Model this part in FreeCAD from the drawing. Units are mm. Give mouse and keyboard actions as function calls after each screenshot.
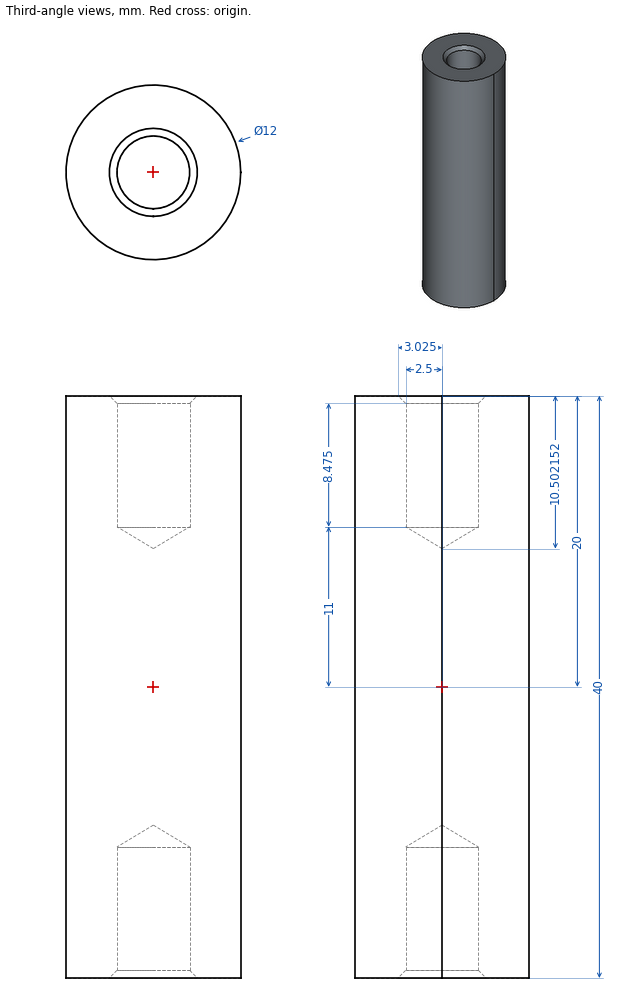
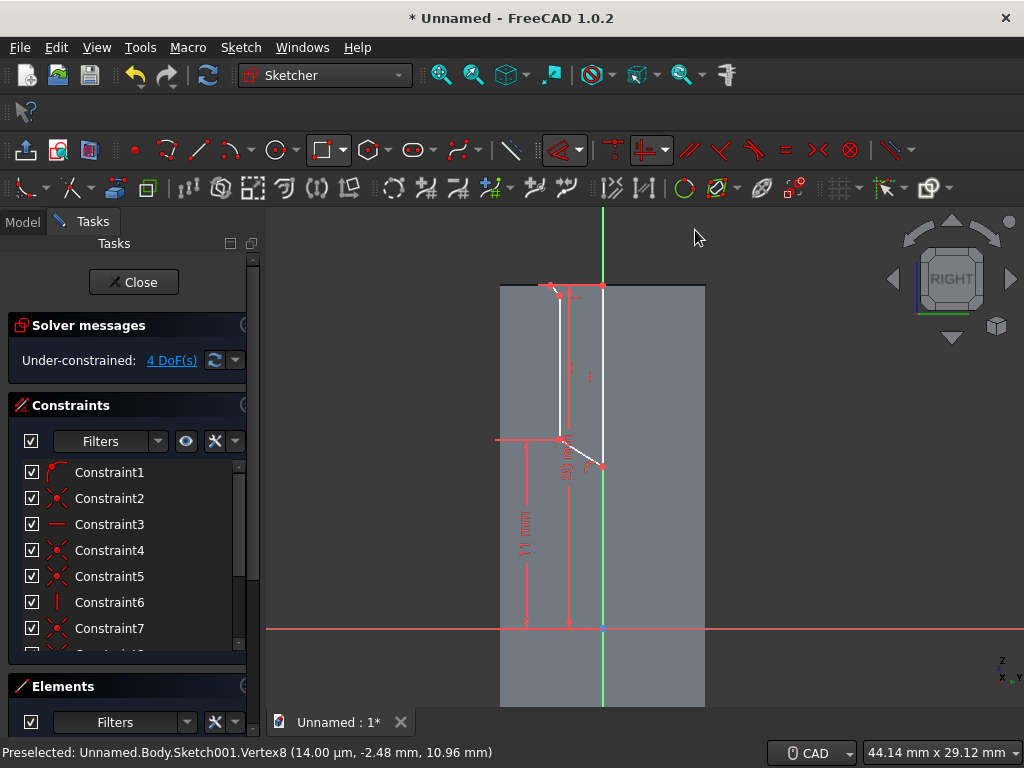
click(560, 295)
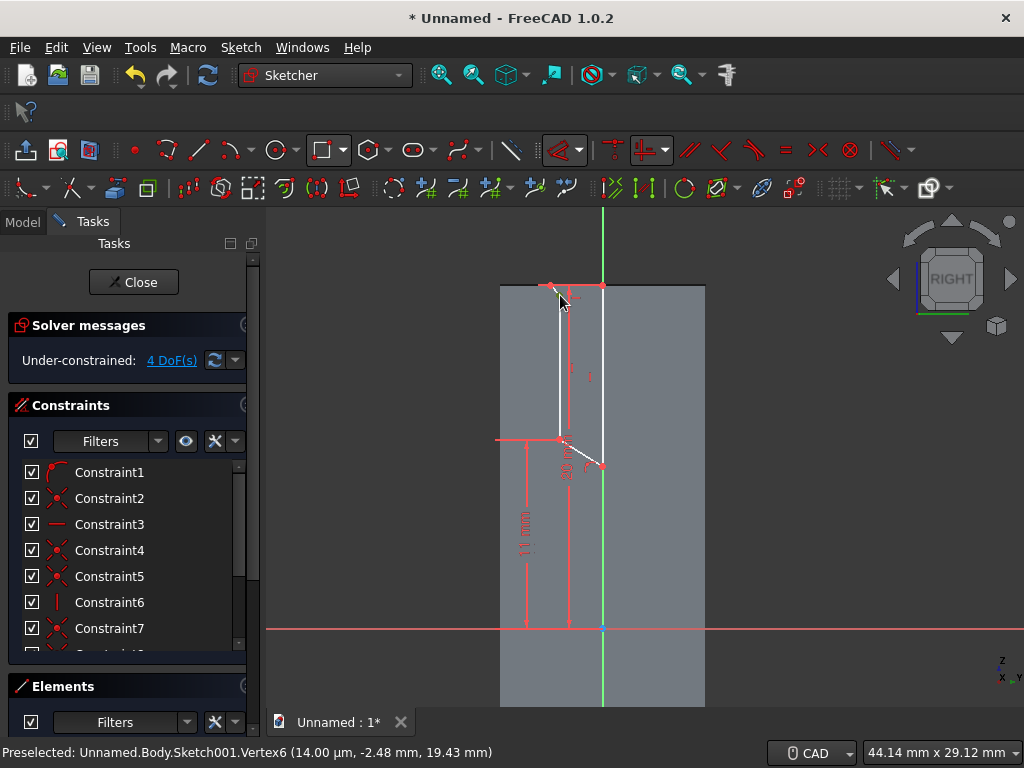
key(l)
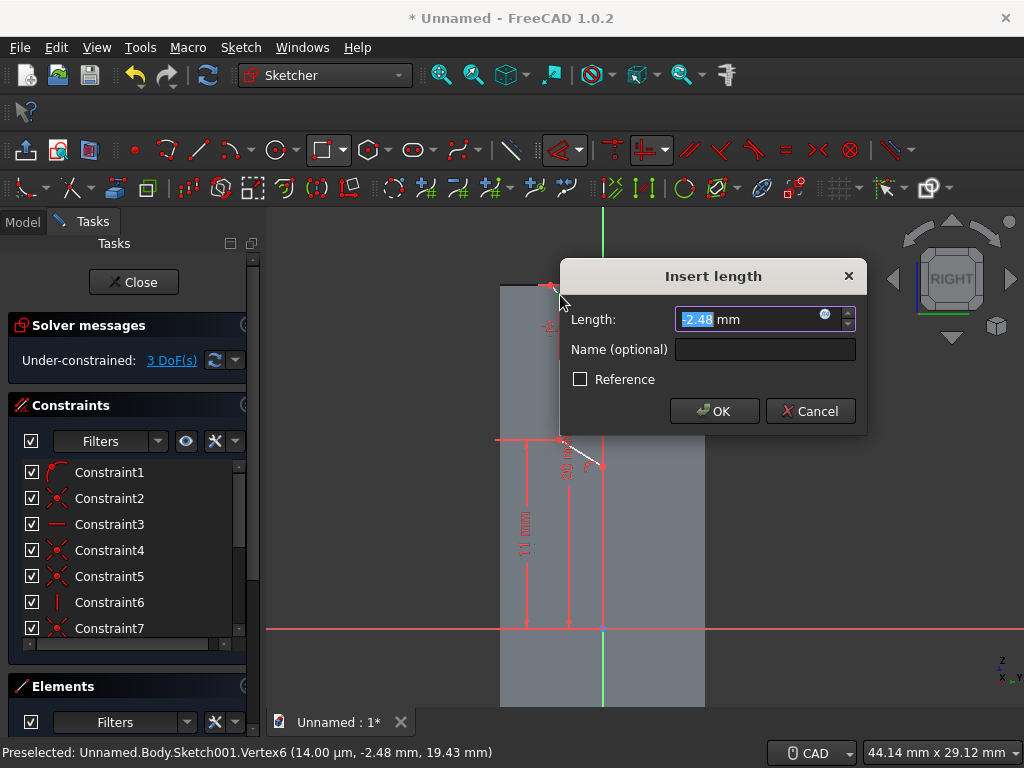
text(-2.5)
key(Return)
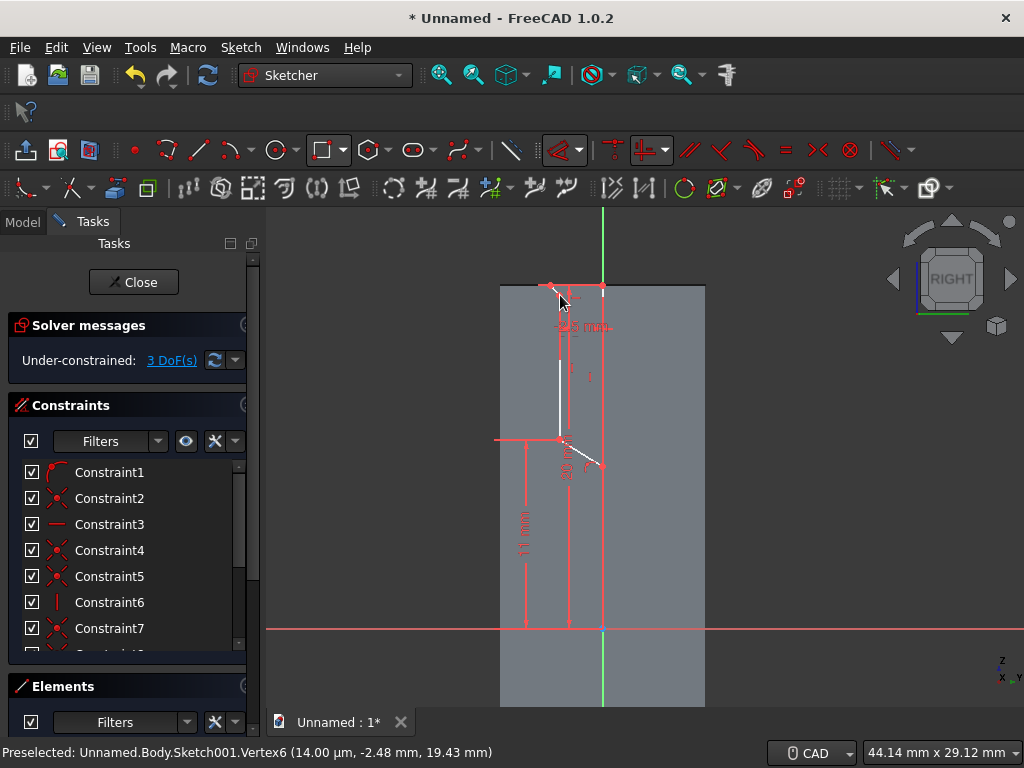
click(587, 285)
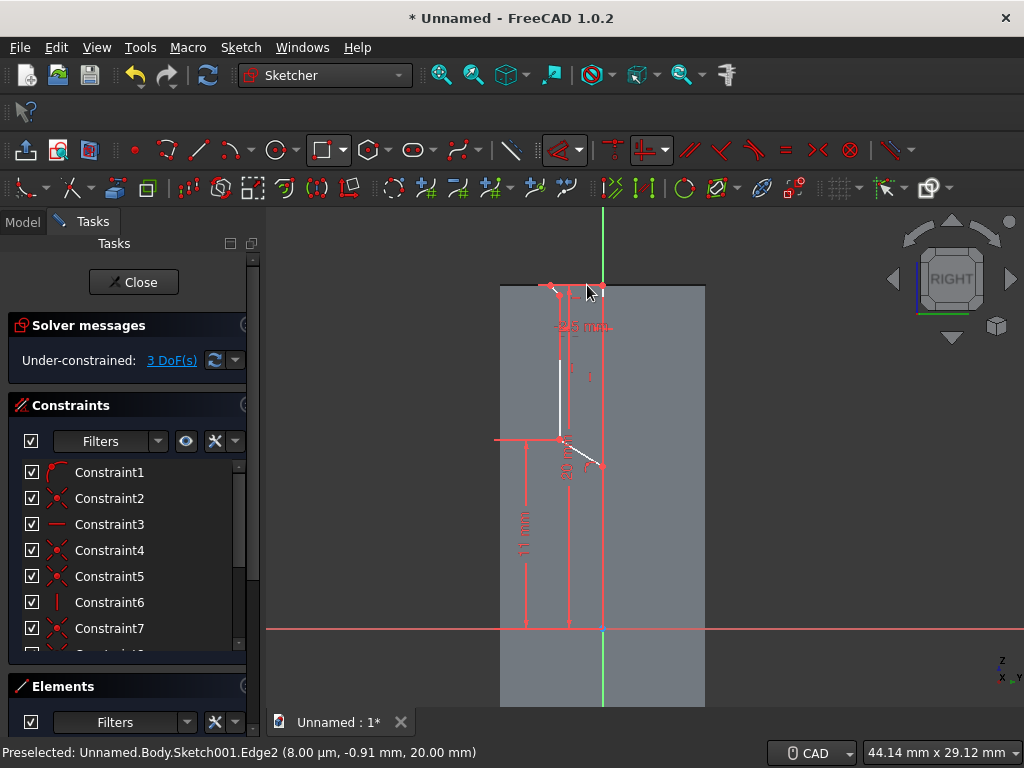
key(l)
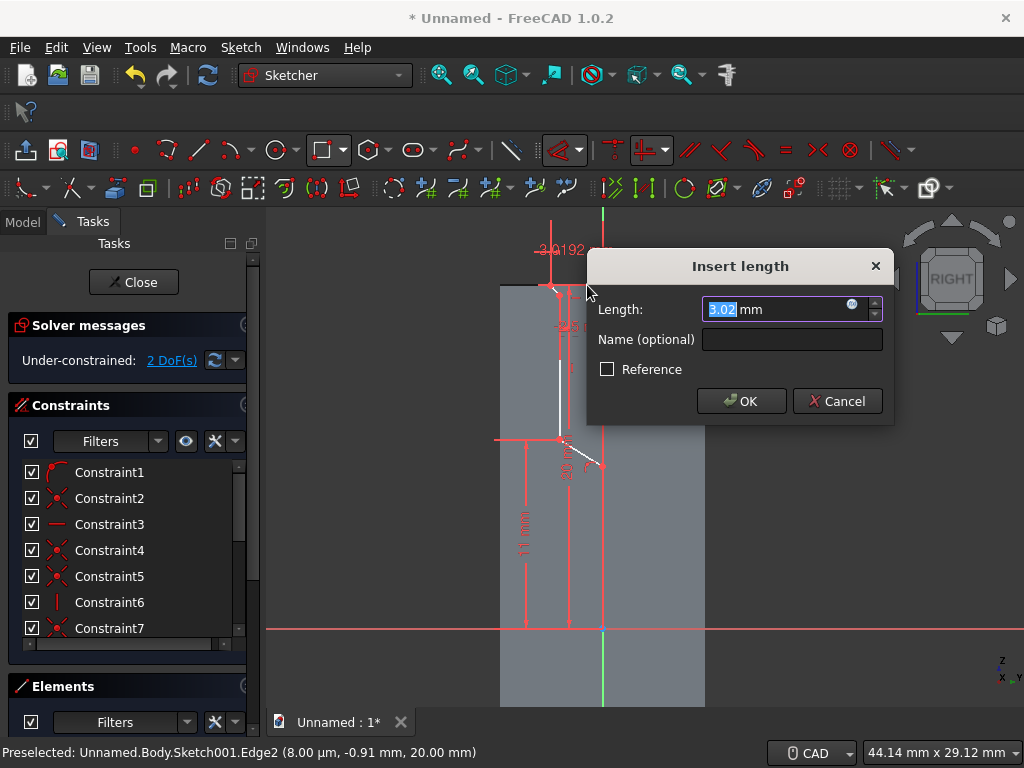
text(3.025)
key(Return)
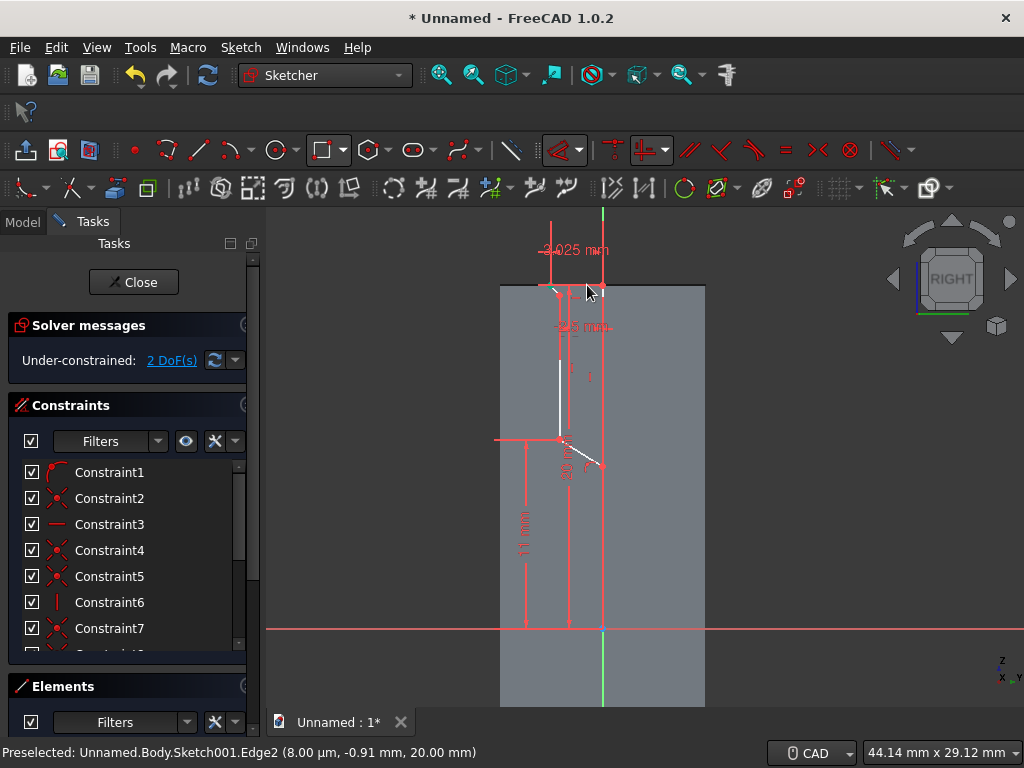
click(560, 339)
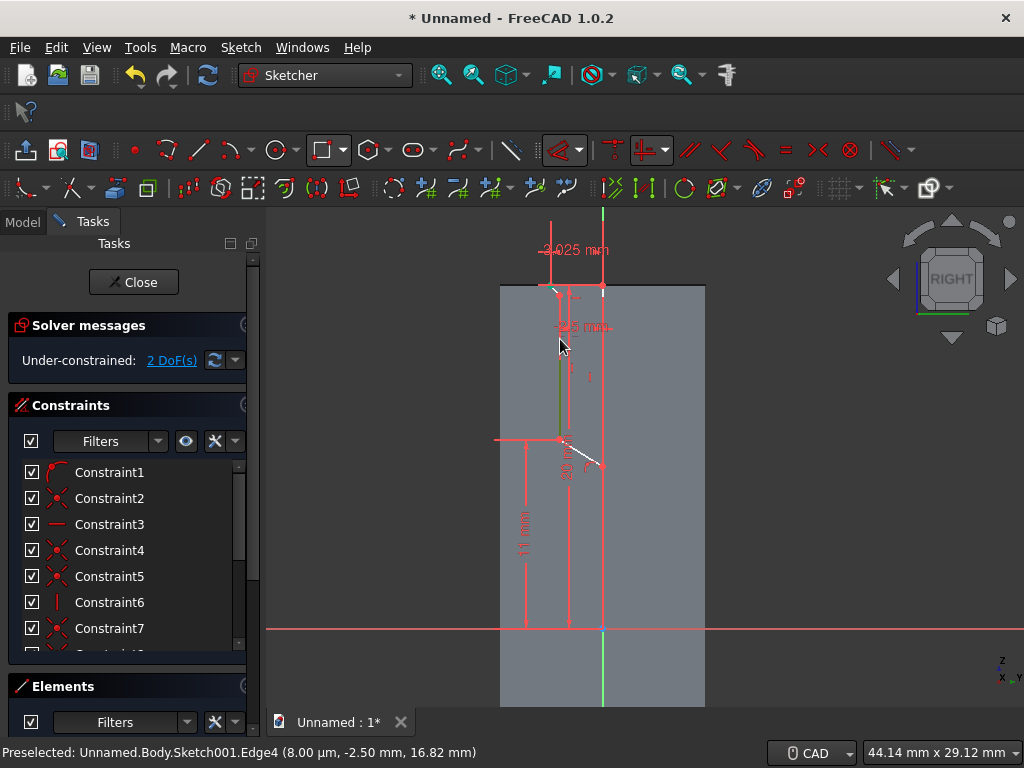
click(582, 150)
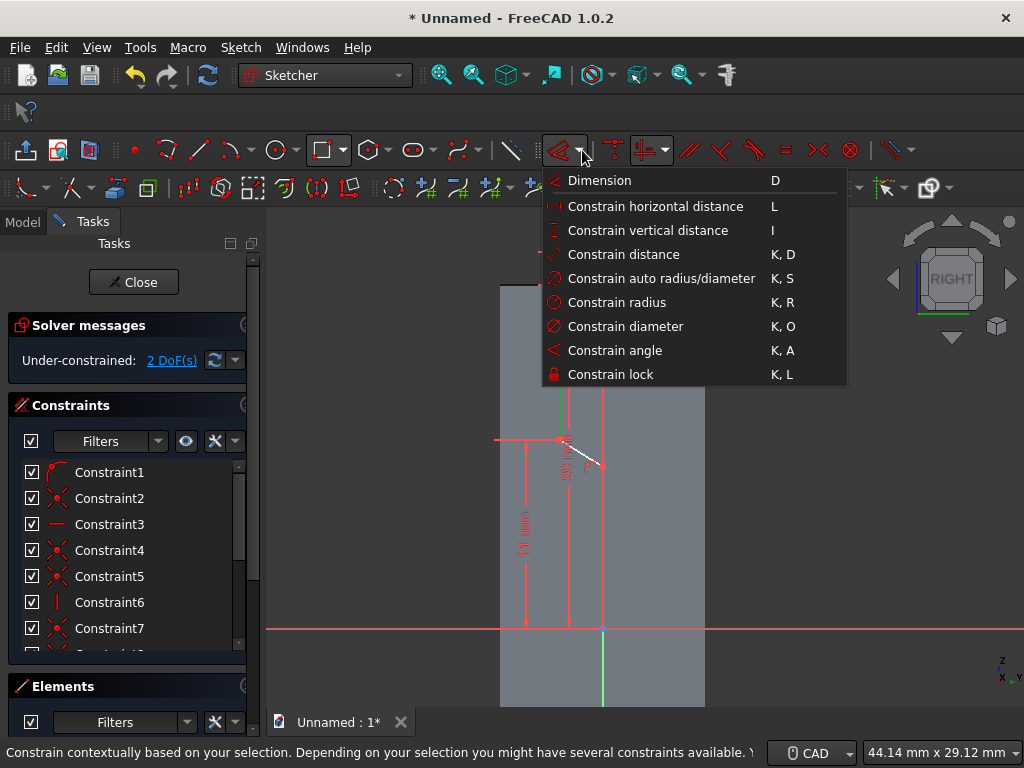
click(695, 230)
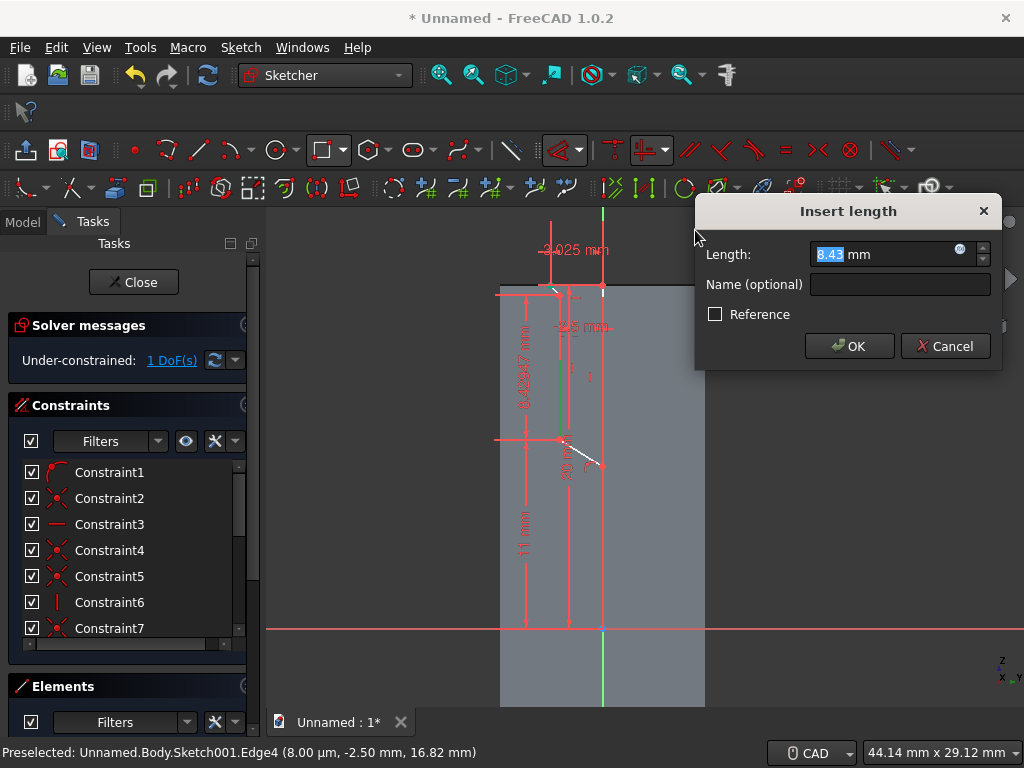
text(8.475)
key(Return)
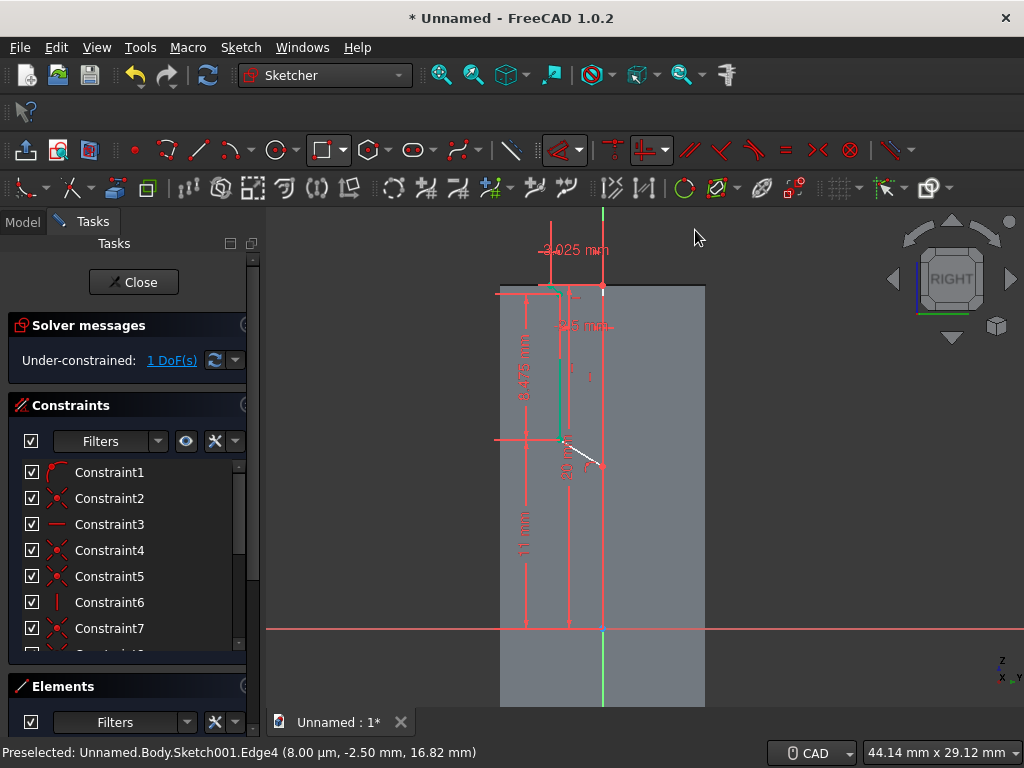
click(603, 412)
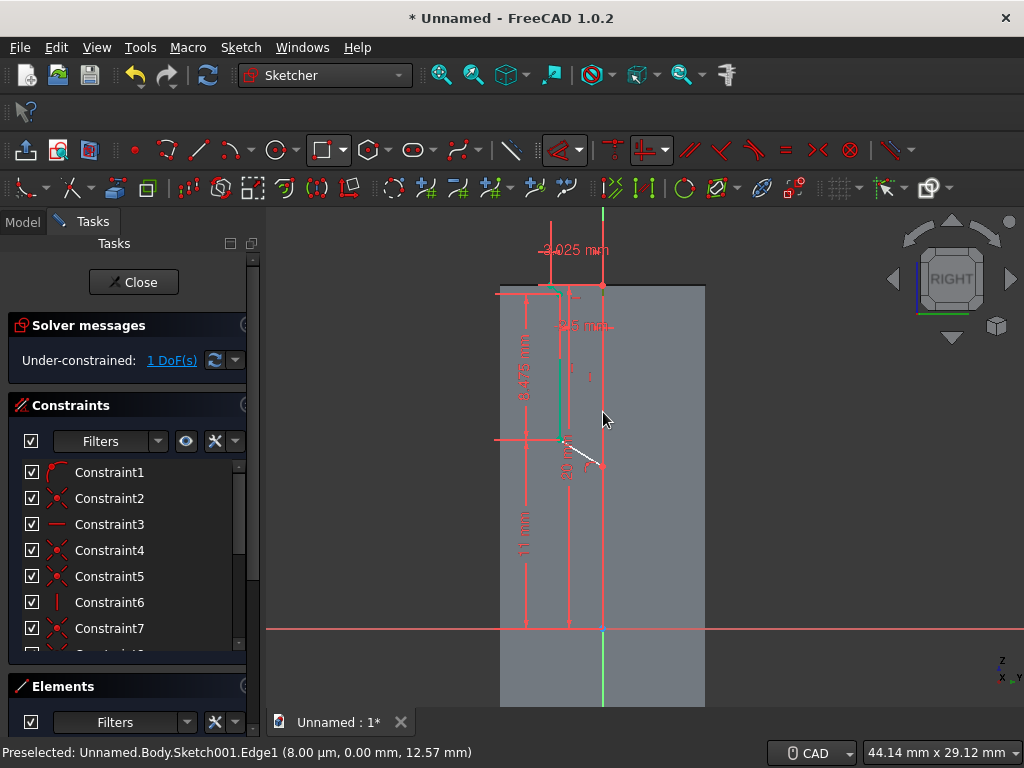
click(582, 150)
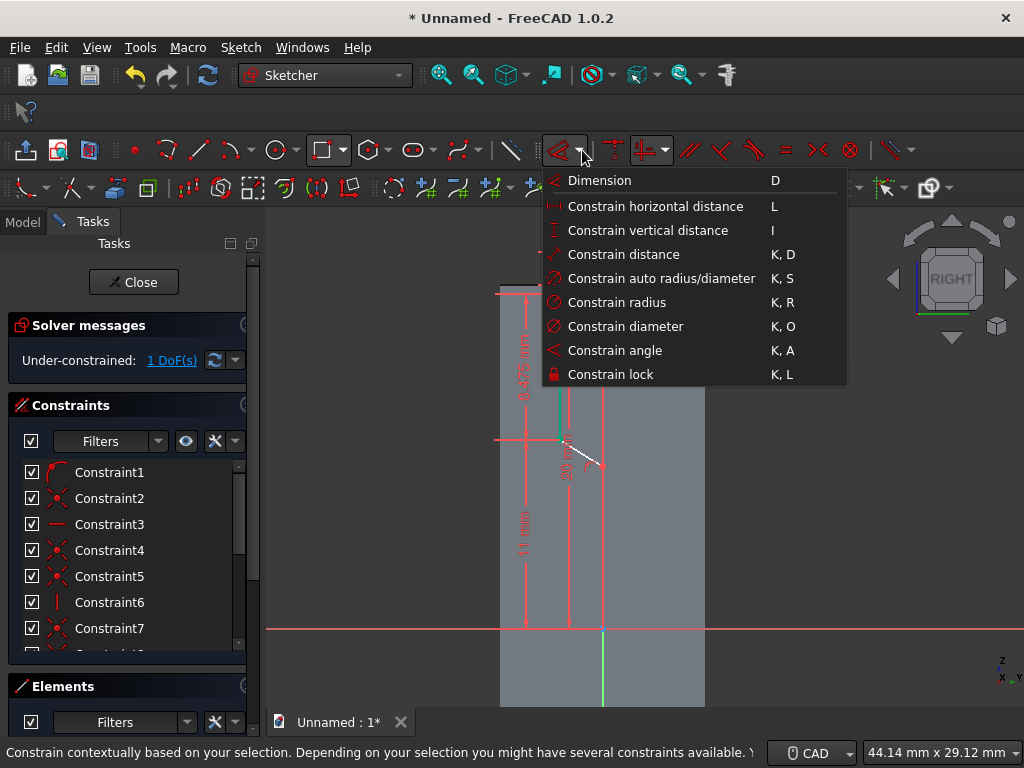
click(695, 230)